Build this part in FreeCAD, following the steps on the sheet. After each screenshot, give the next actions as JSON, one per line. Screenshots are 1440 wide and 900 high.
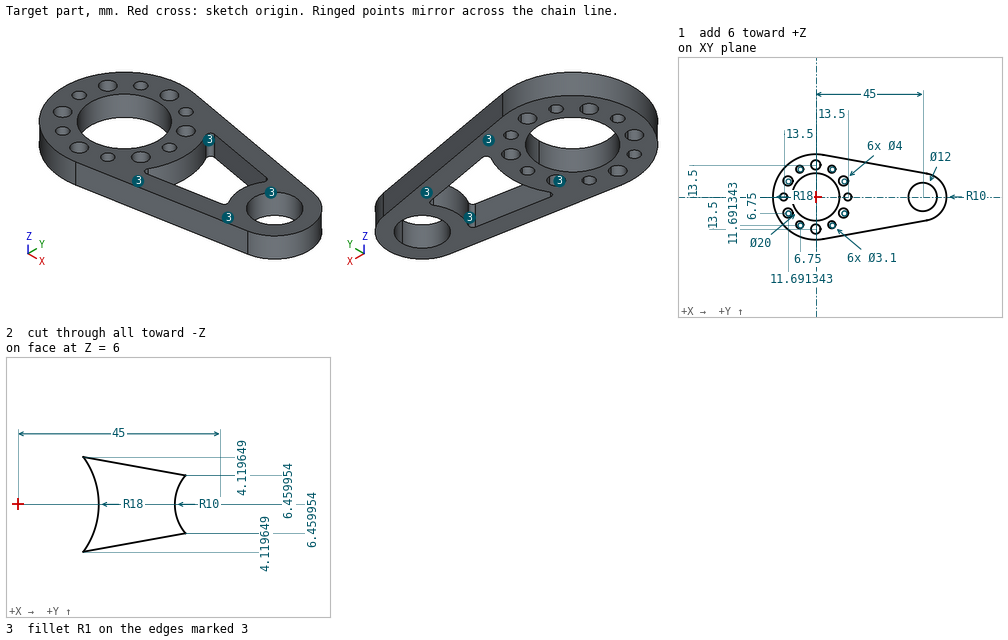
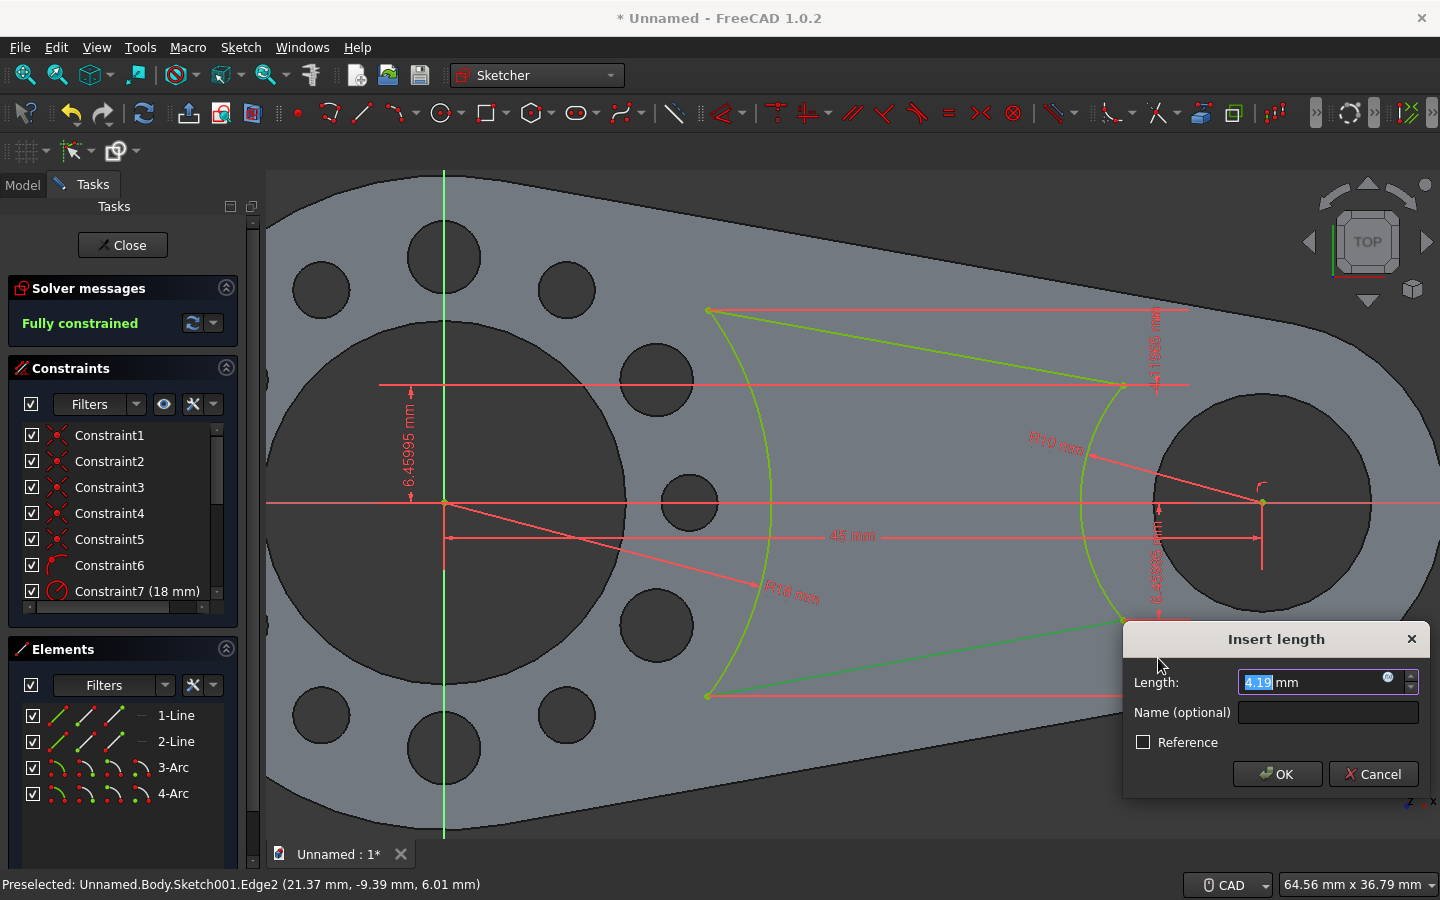
{"action": "type", "text": "4.119649"}
{"action": "key", "text": "Return"}
{"action": "key", "text": "Escape"}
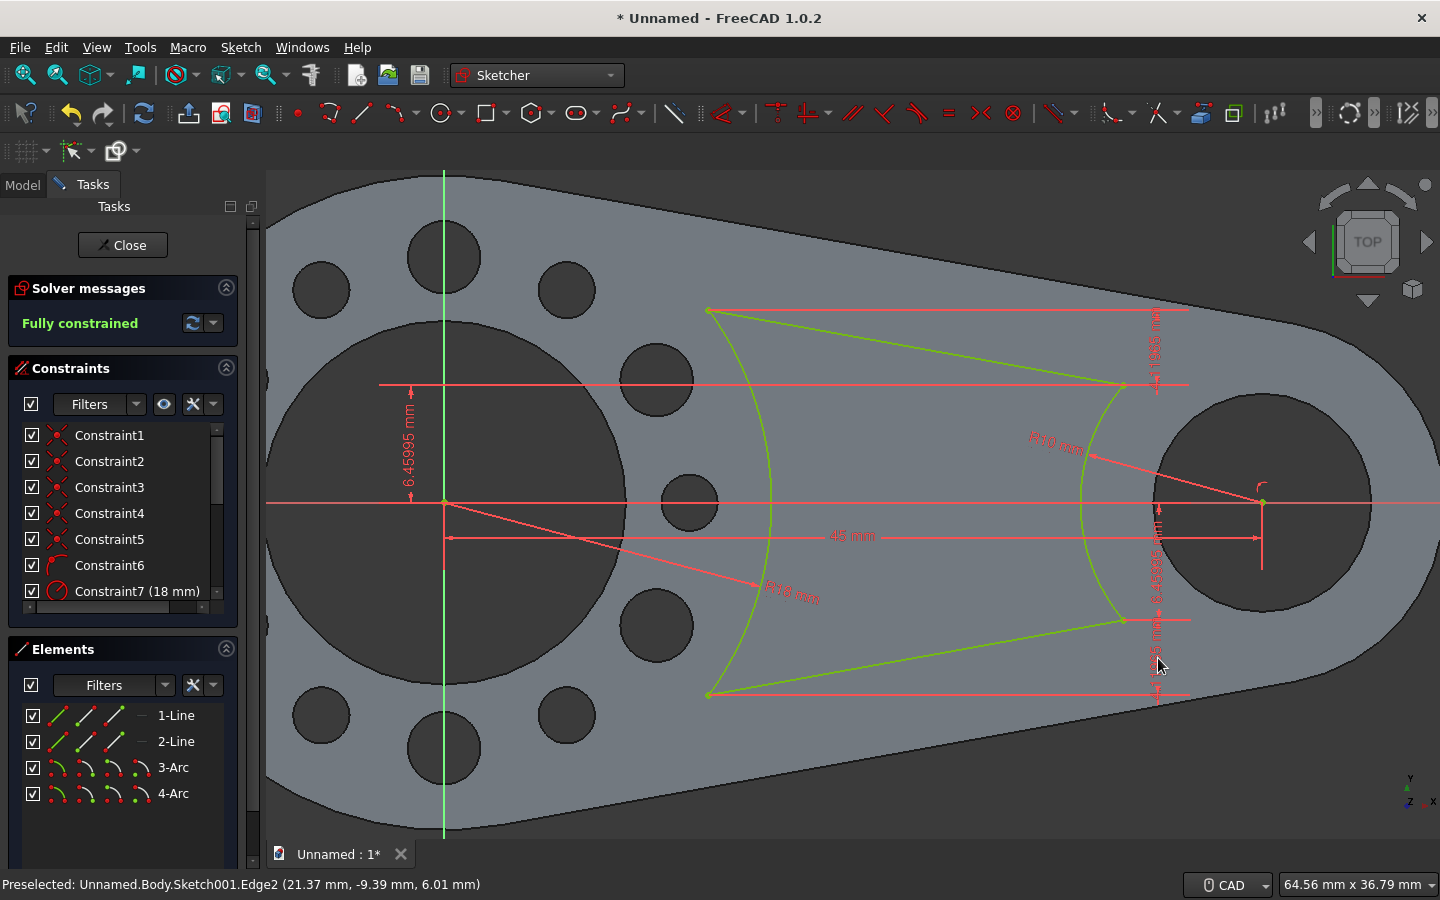
{"action": "left_click", "coordinate": [123, 245]}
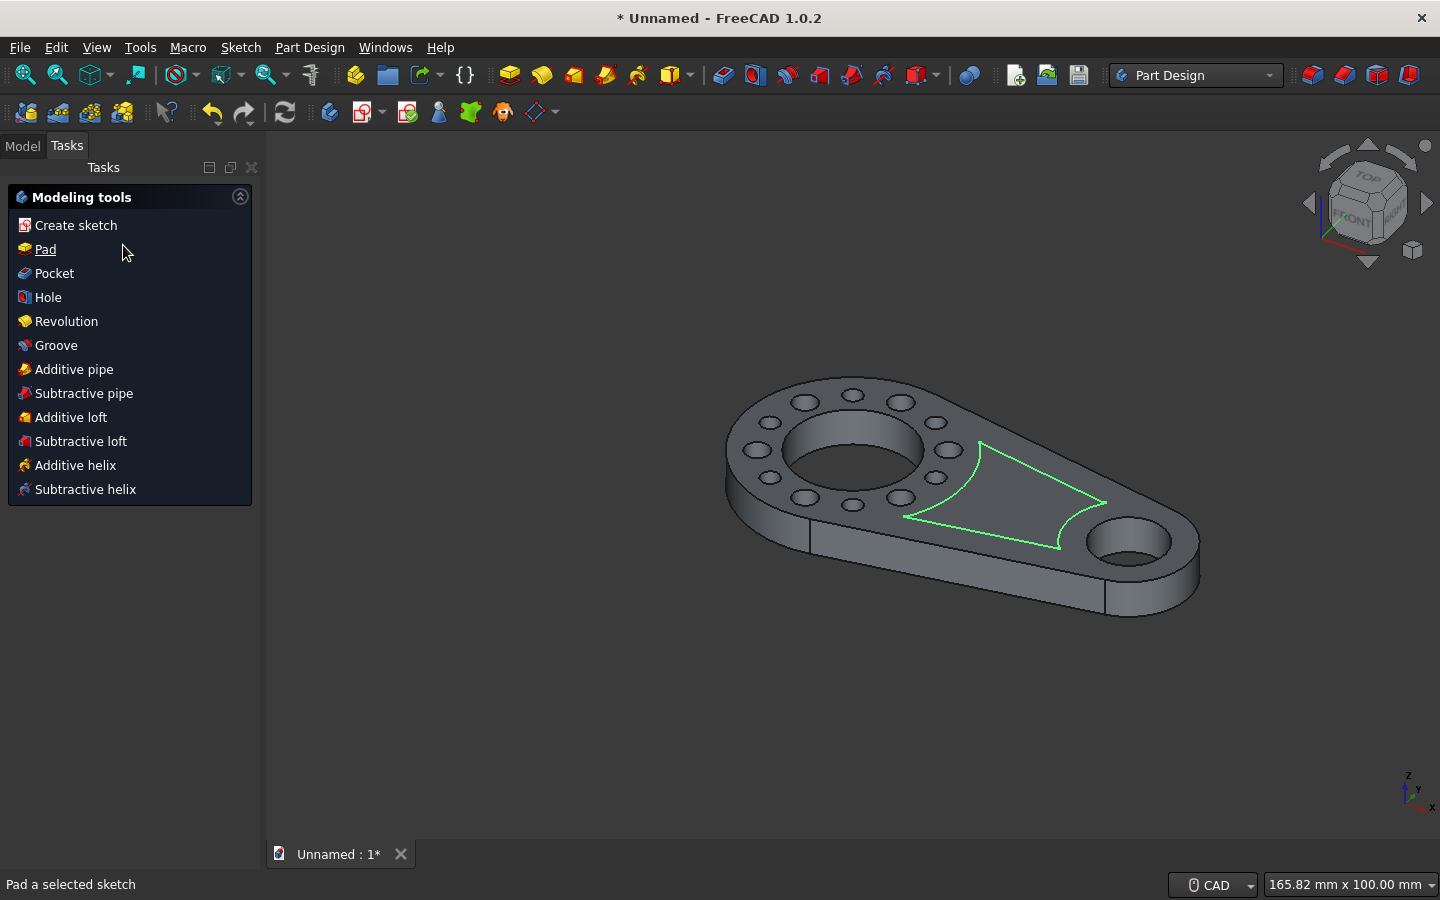
{"action": "left_click", "coordinate": [724, 76]}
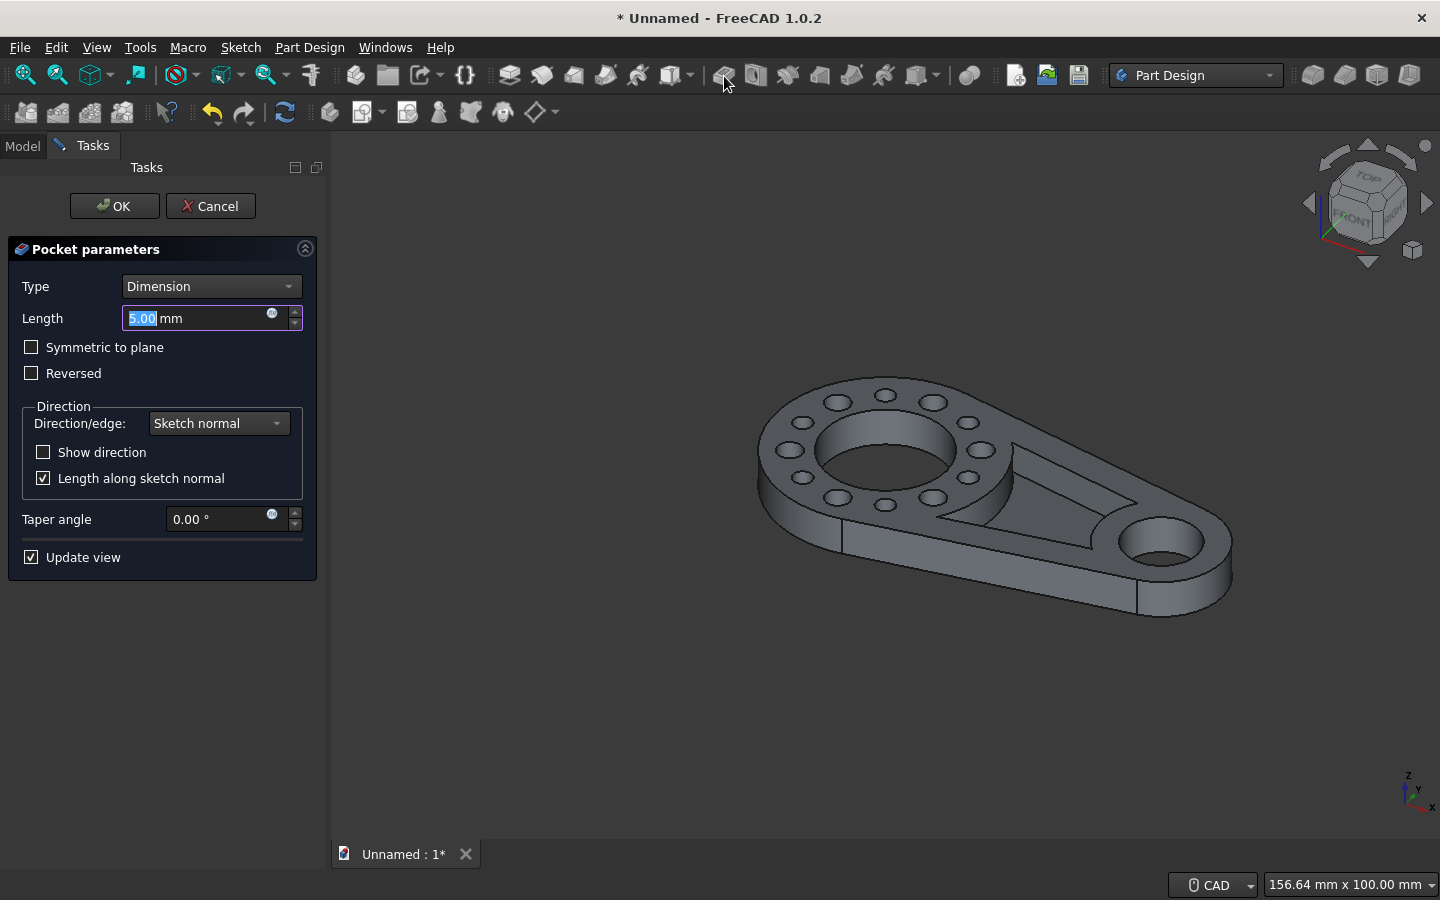
{"action": "left_click", "coordinate": [212, 286]}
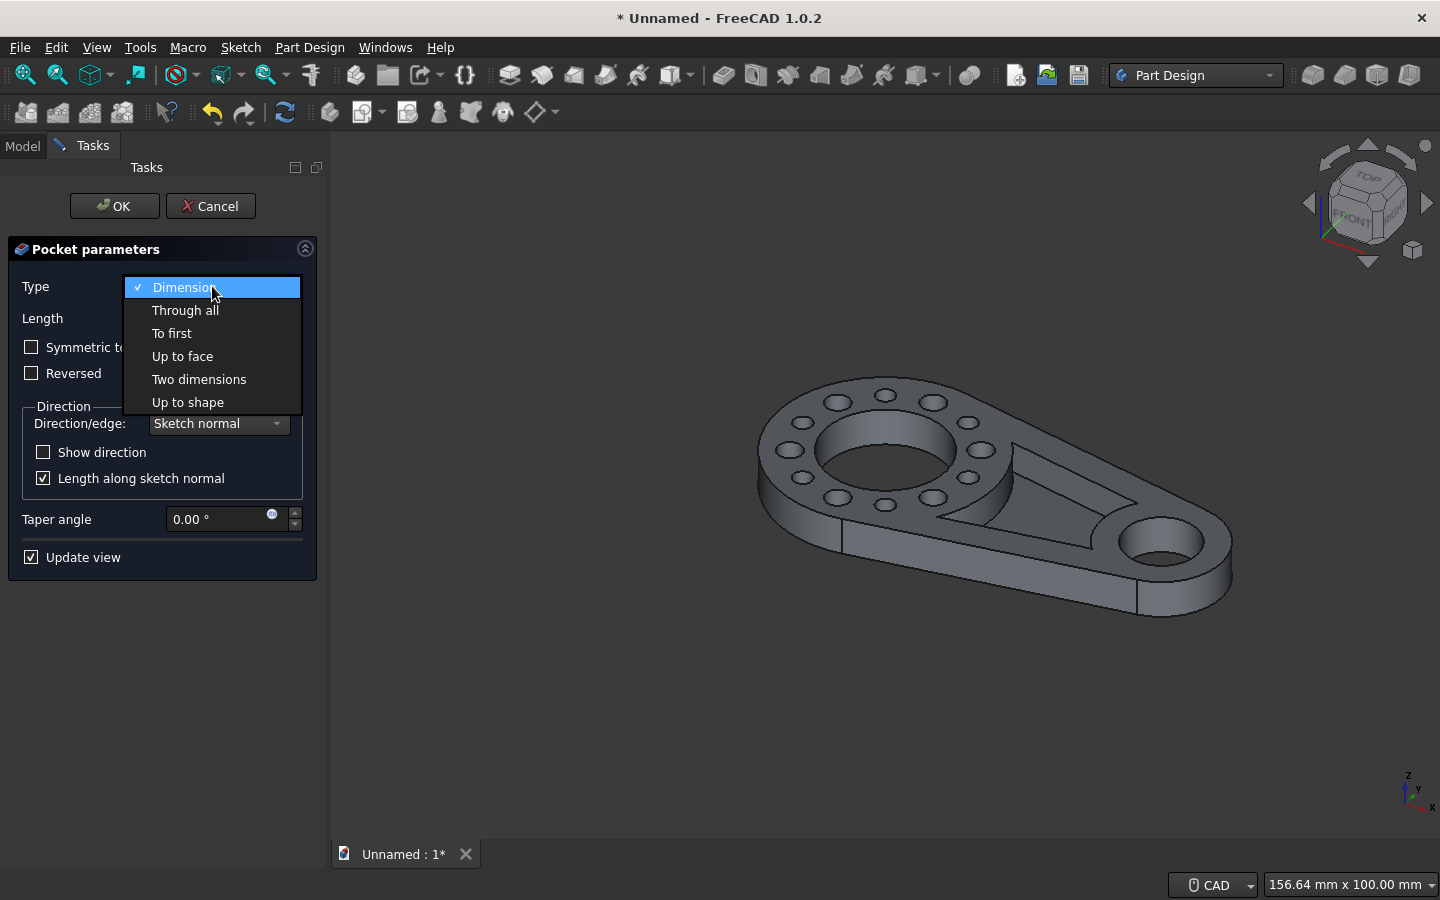
{"action": "left_click", "coordinate": [212, 310]}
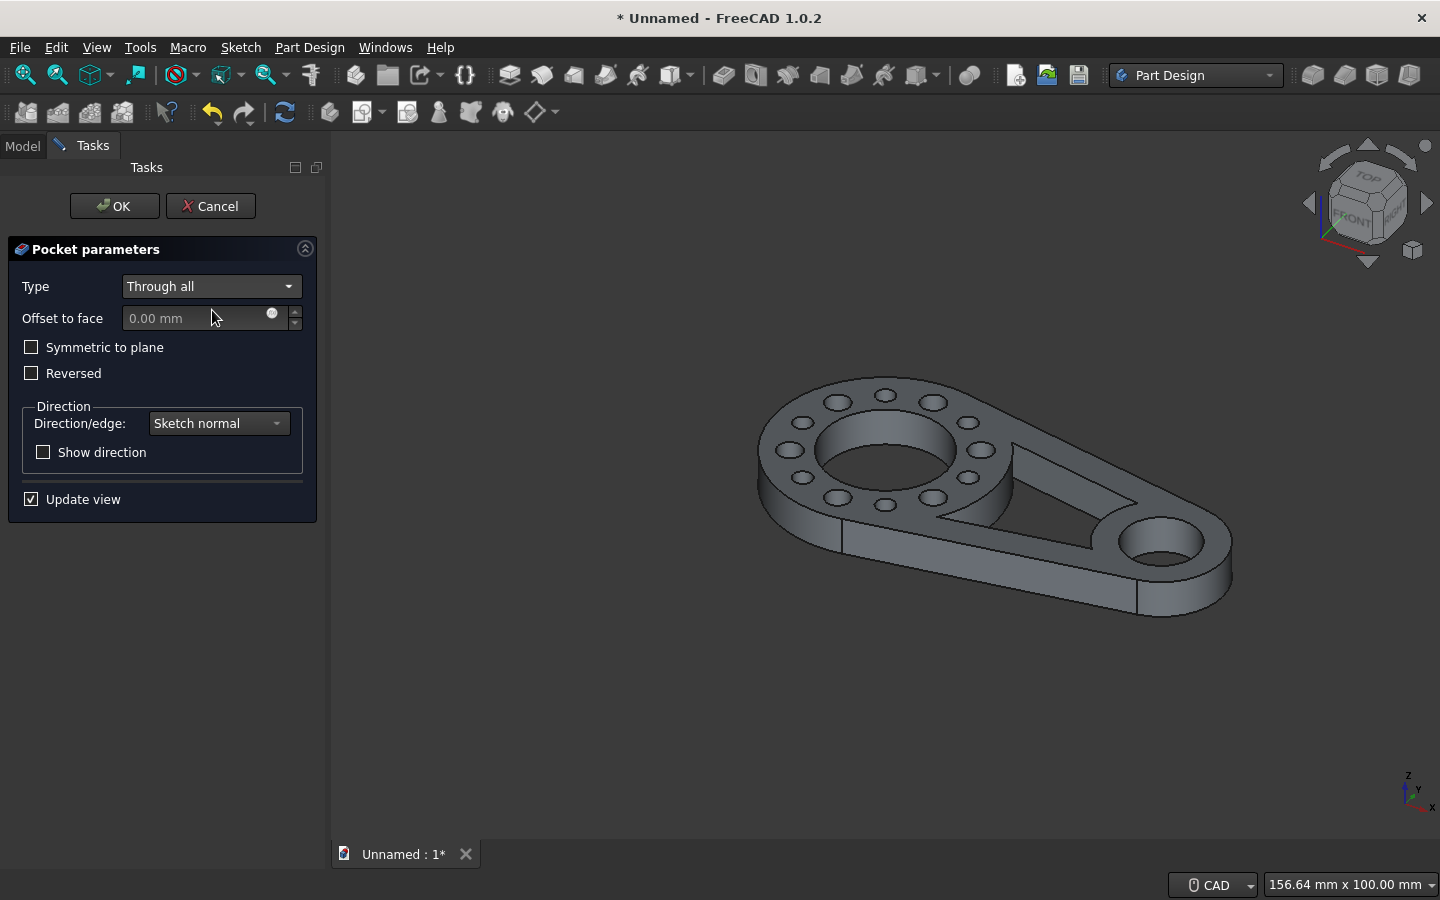
{"action": "left_click", "coordinate": [115, 206]}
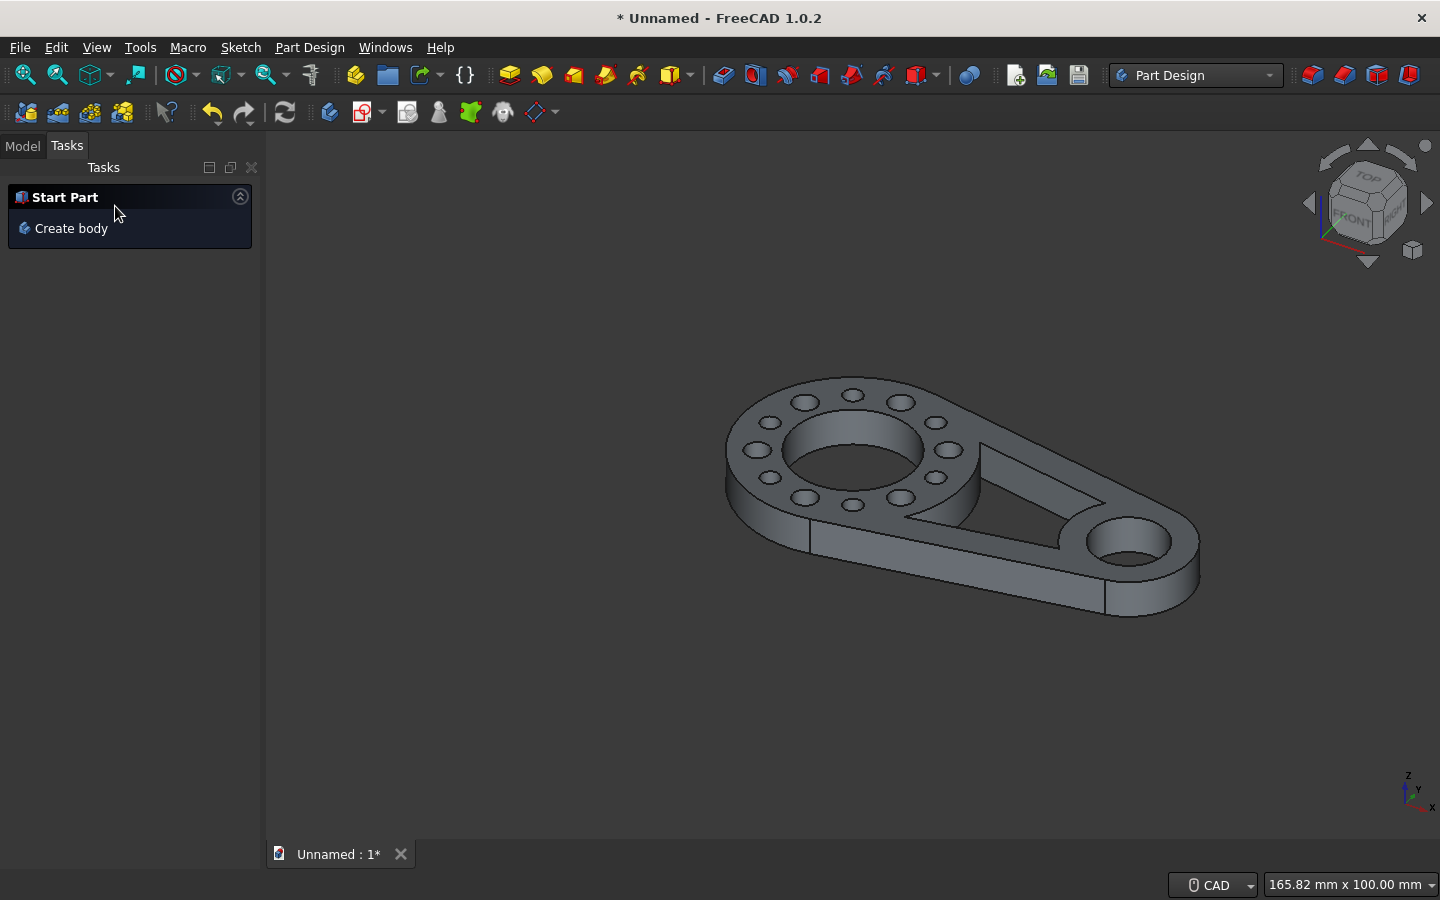
{"action": "key", "text": "0"}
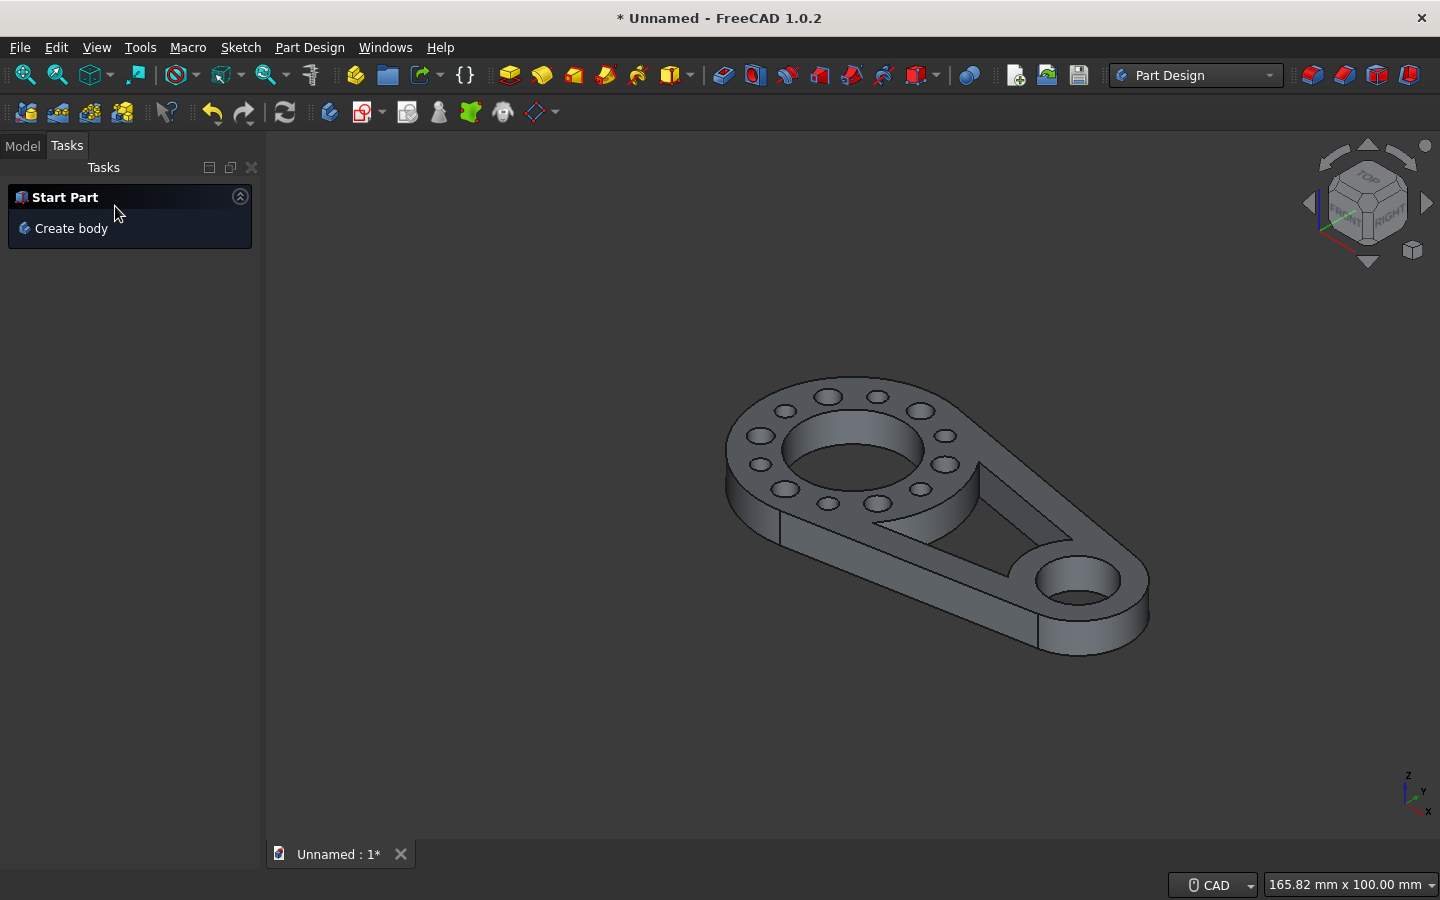
{"action": "key", "text": "2"}